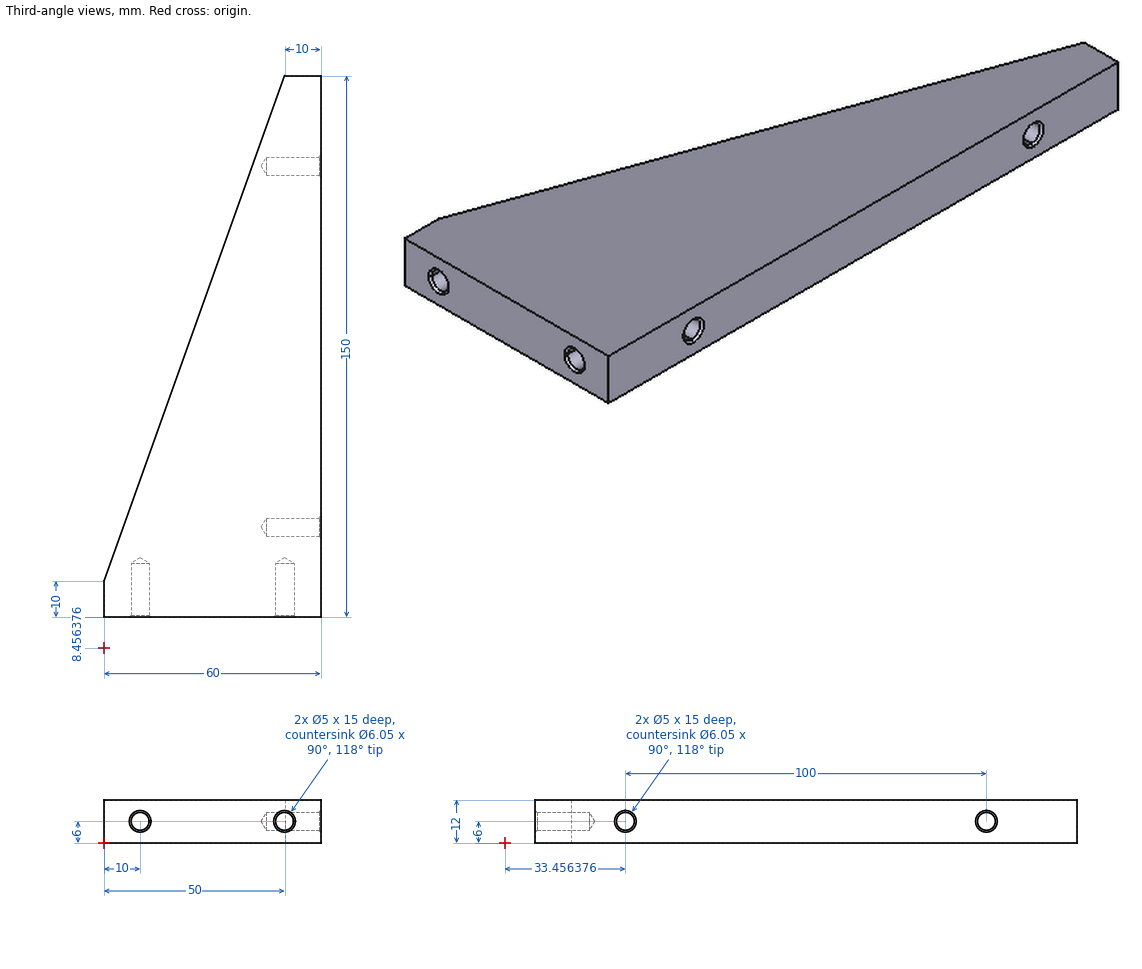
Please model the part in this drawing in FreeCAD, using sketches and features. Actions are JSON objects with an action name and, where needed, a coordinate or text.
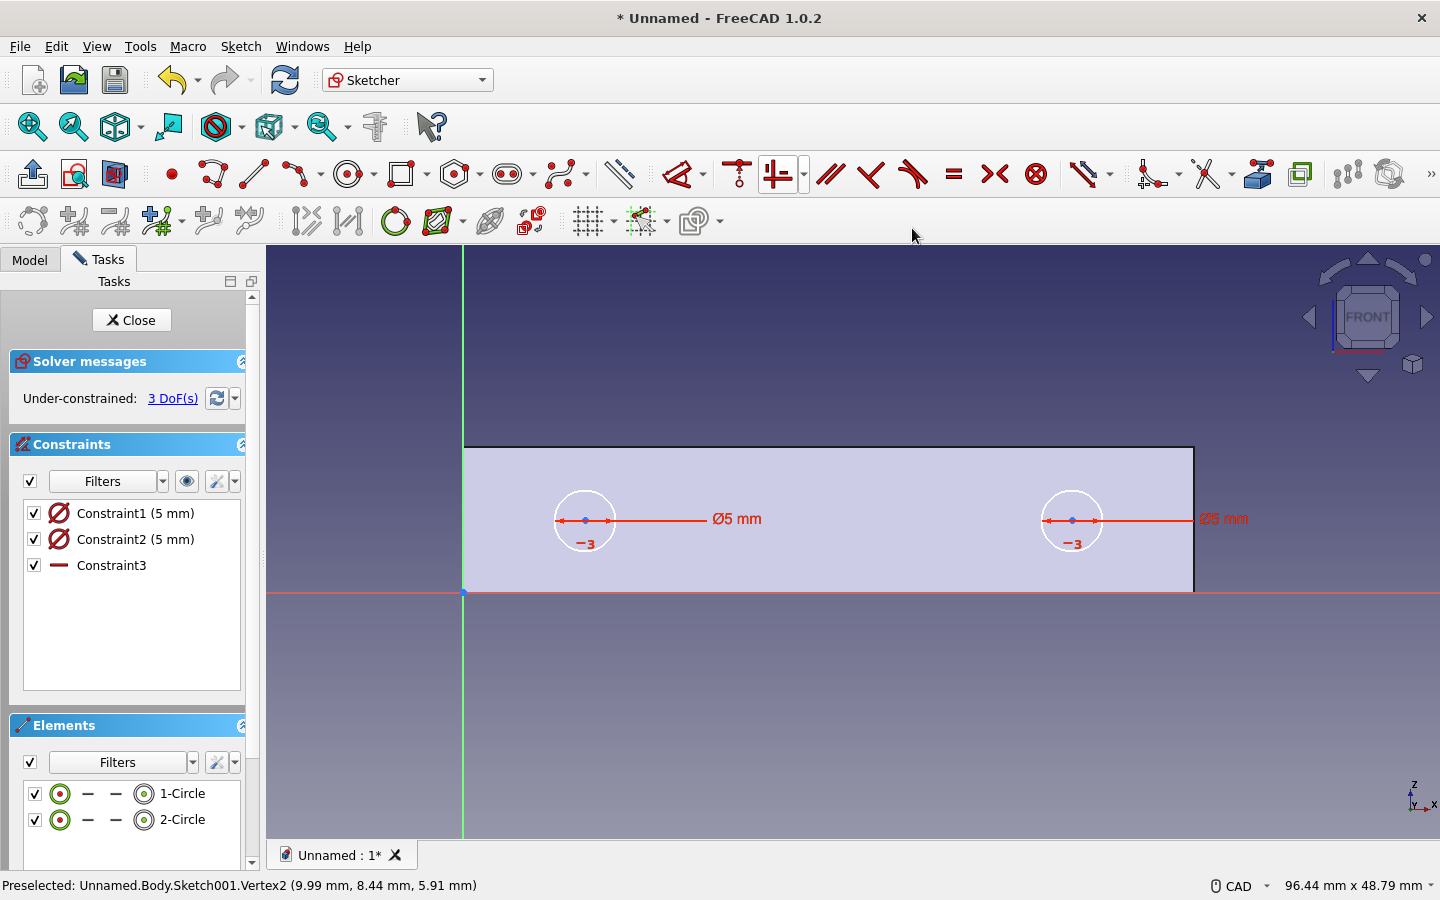
{"action": "left_click", "coordinate": [676, 174]}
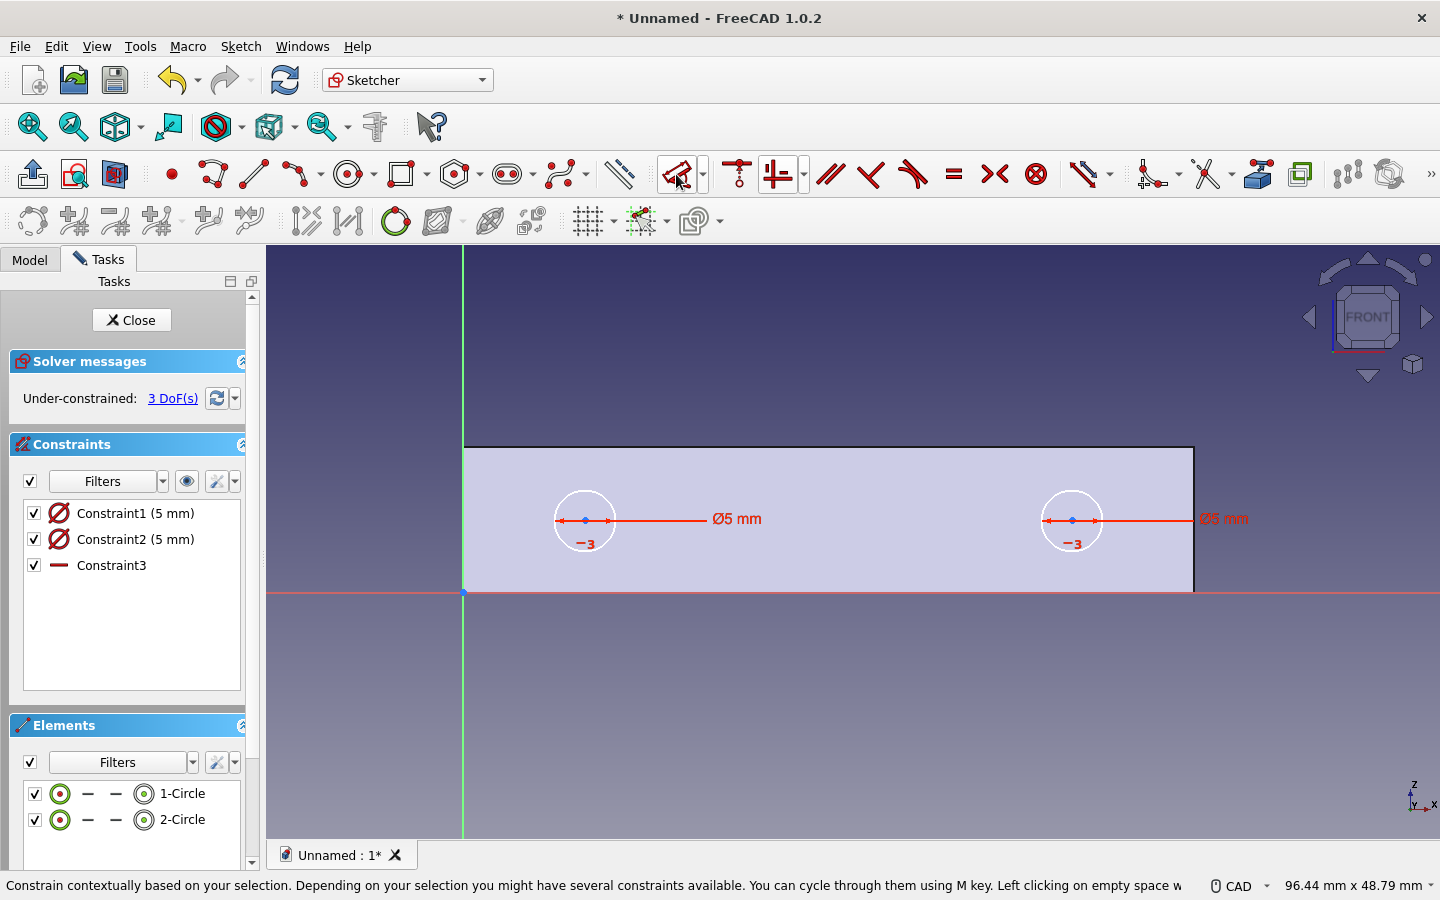
{"action": "left_click", "coordinate": [1072, 521]}
{"action": "left_click", "coordinate": [429, 557]}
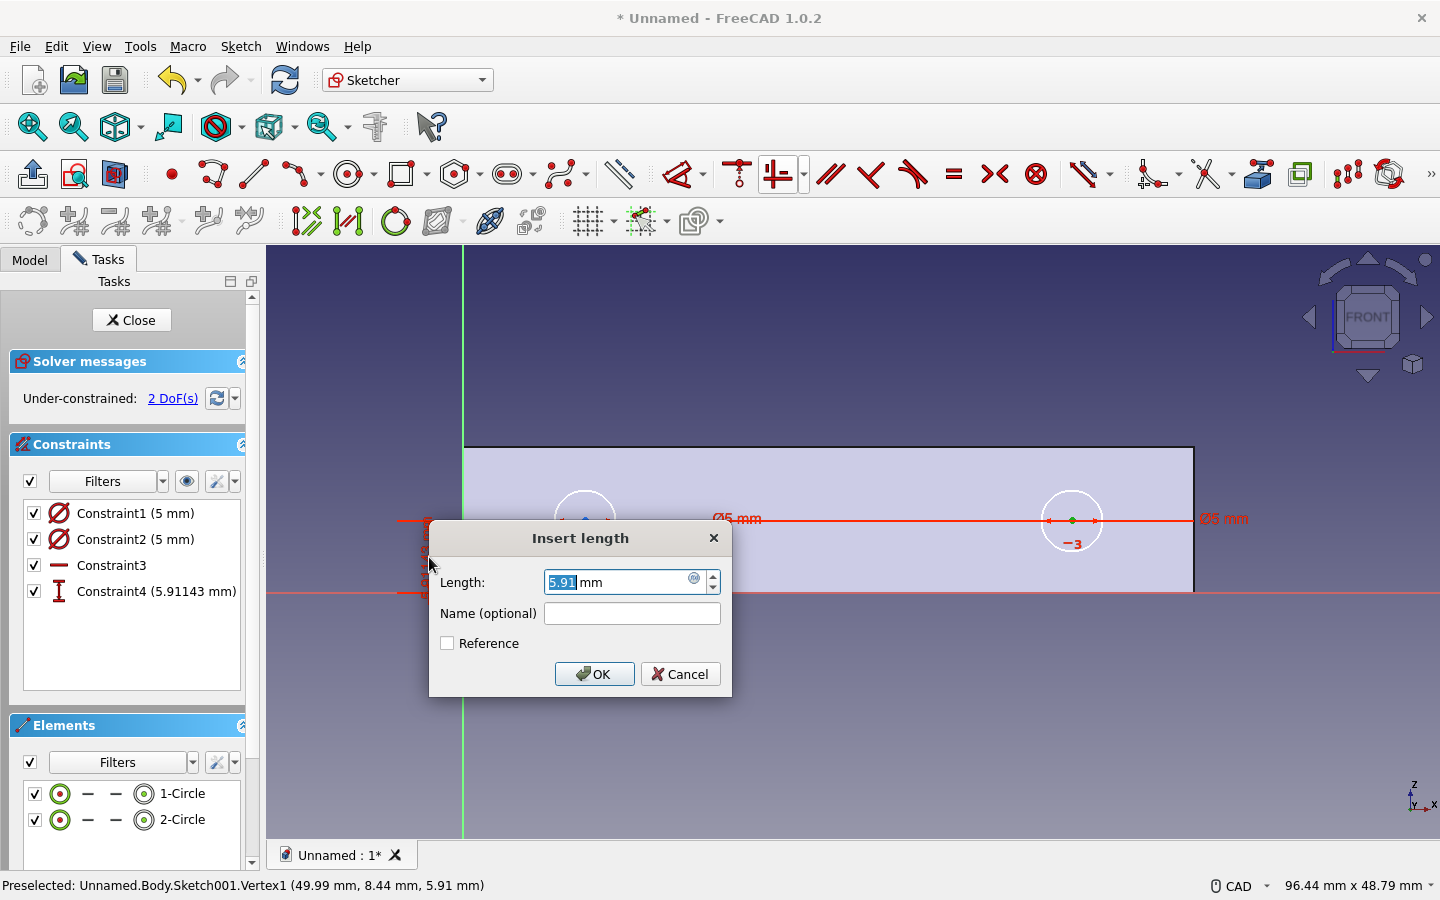
{"action": "type", "text": "6"}
{"action": "key", "text": "Return"}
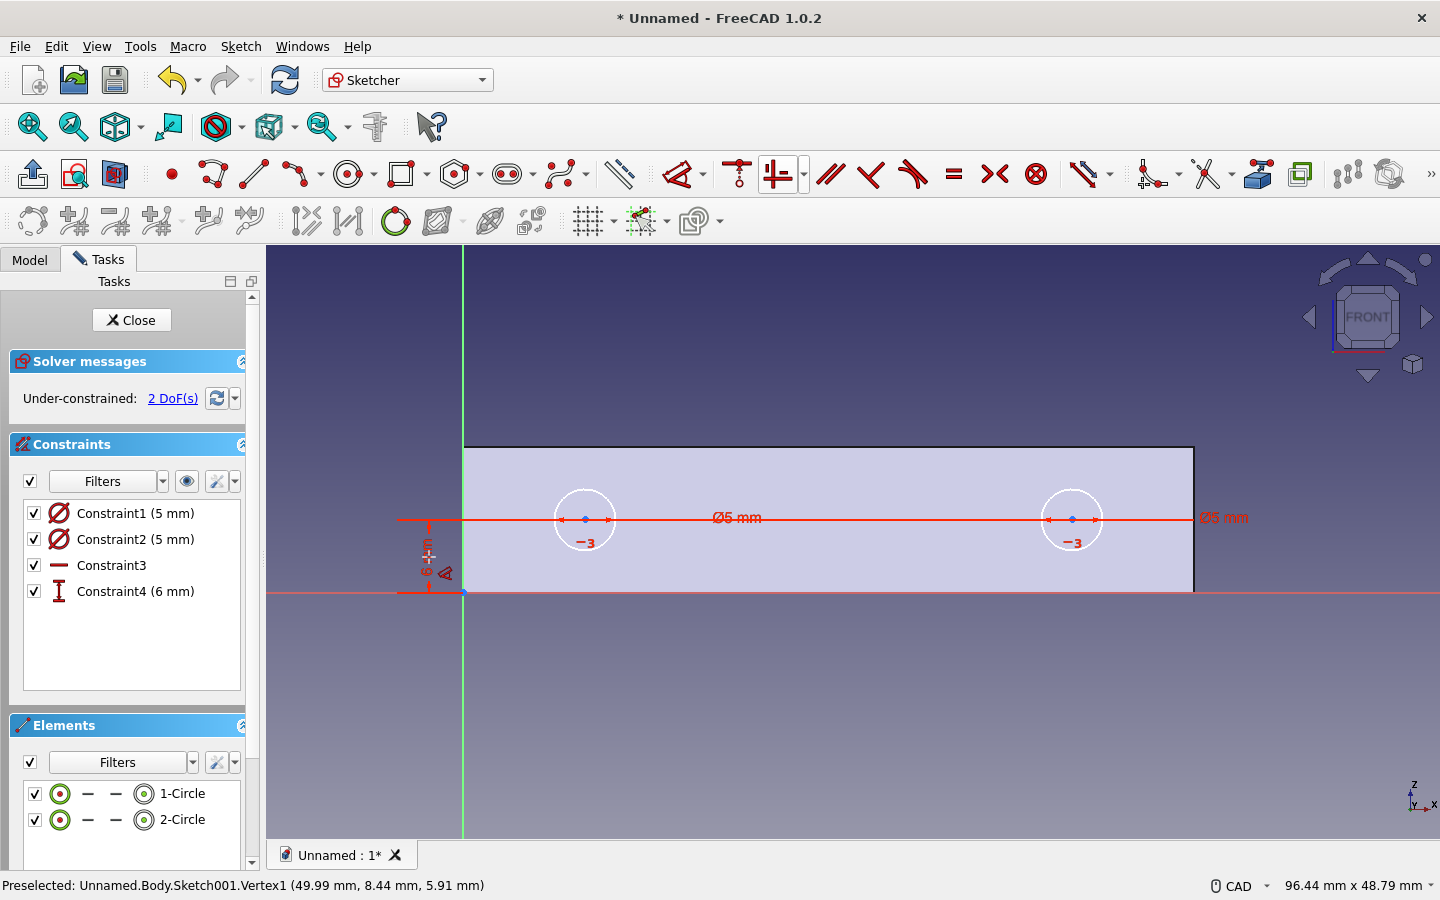
{"action": "left_click", "coordinate": [1072, 520]}
{"action": "left_click", "coordinate": [768, 627]}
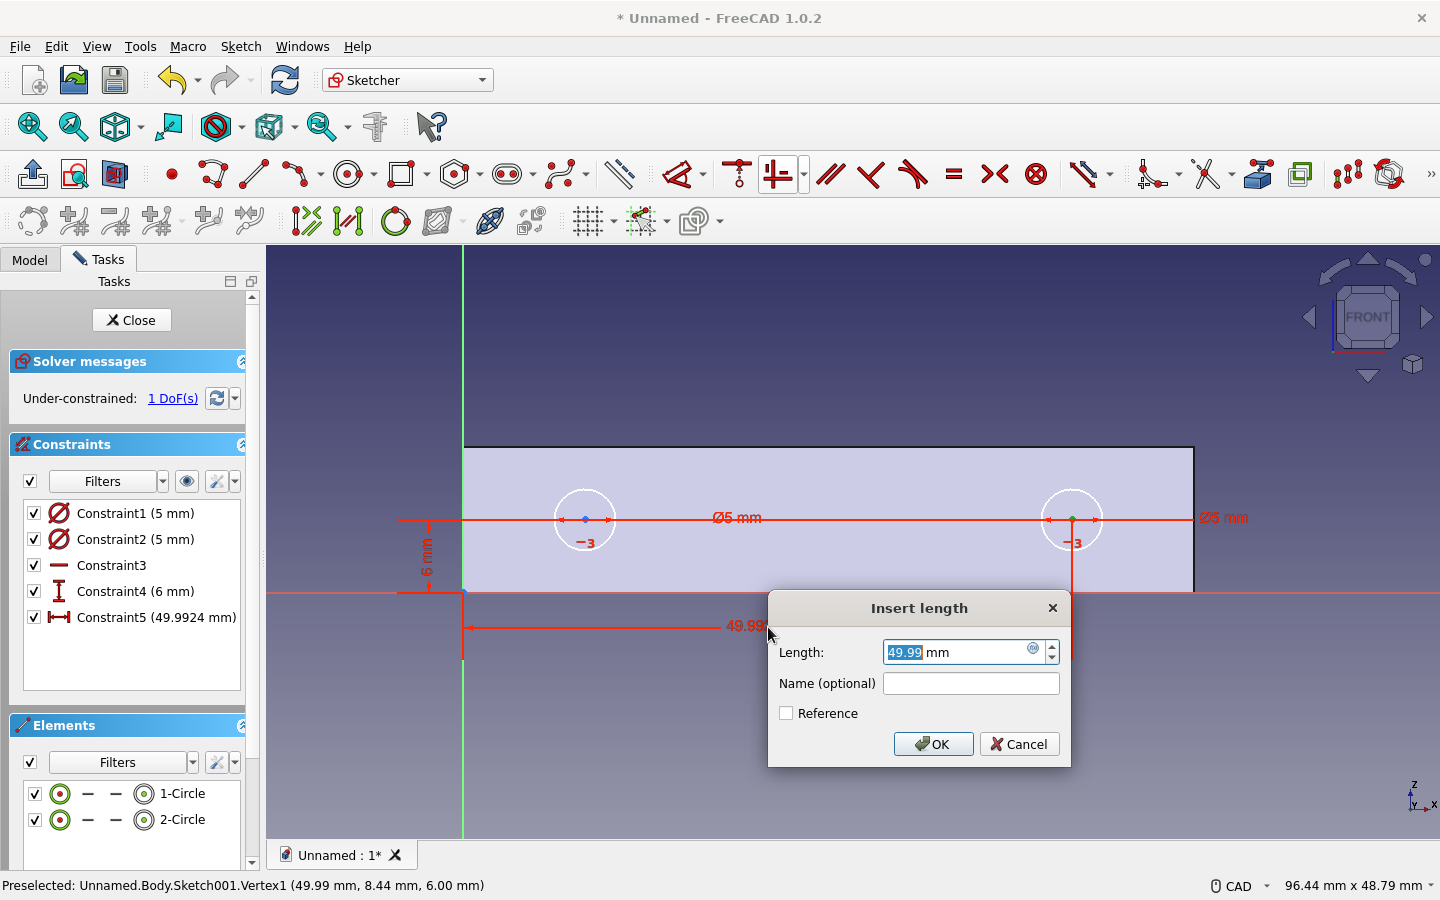
{"action": "type", "text": "50"}
{"action": "key", "text": "Return"}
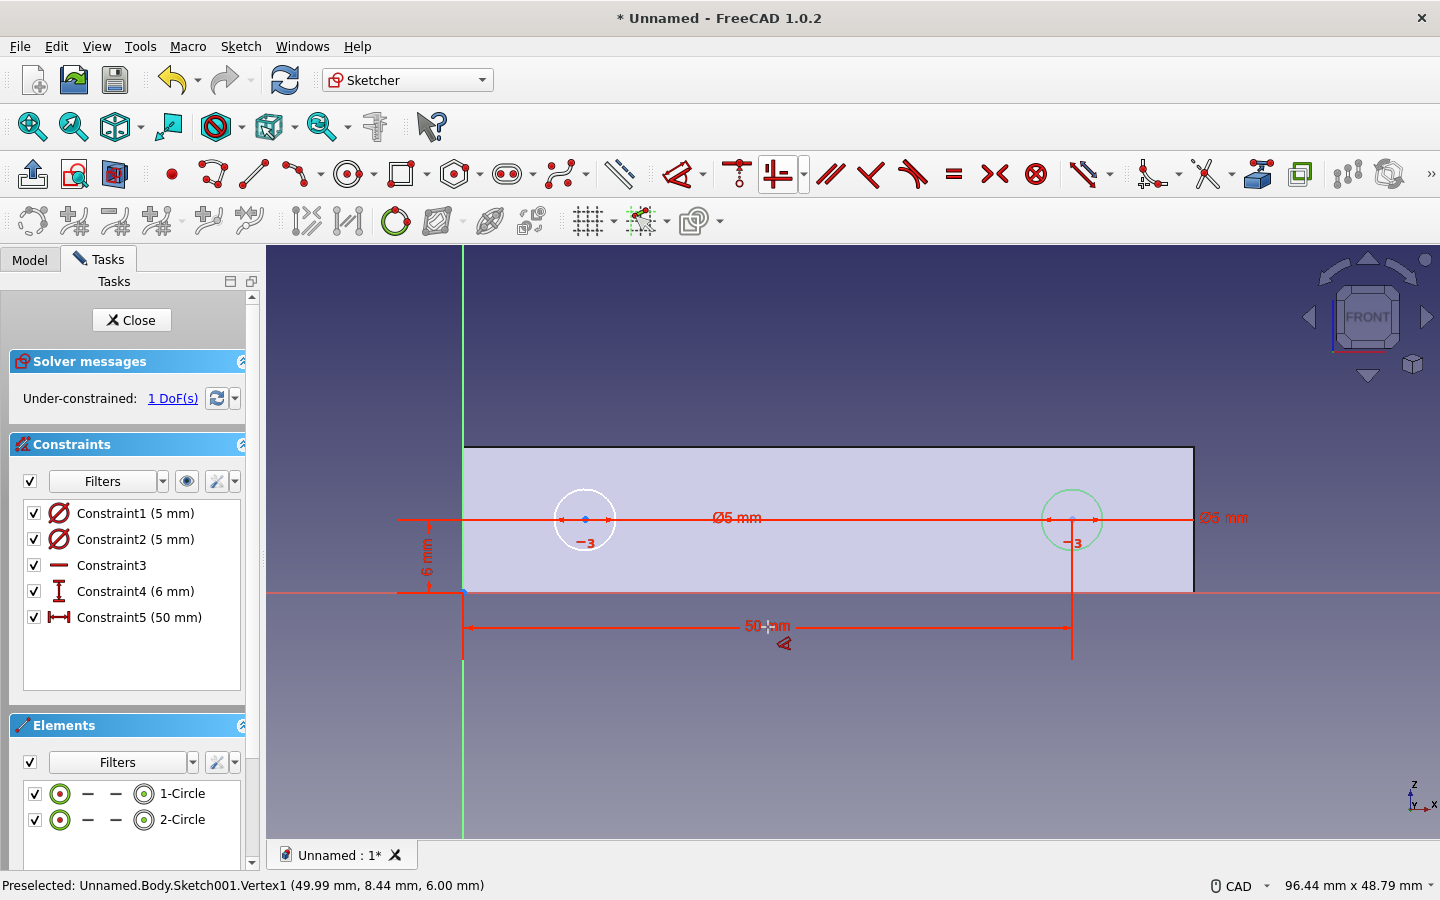
{"action": "left_click", "coordinate": [585, 520]}
{"action": "left_click", "coordinate": [524, 627]}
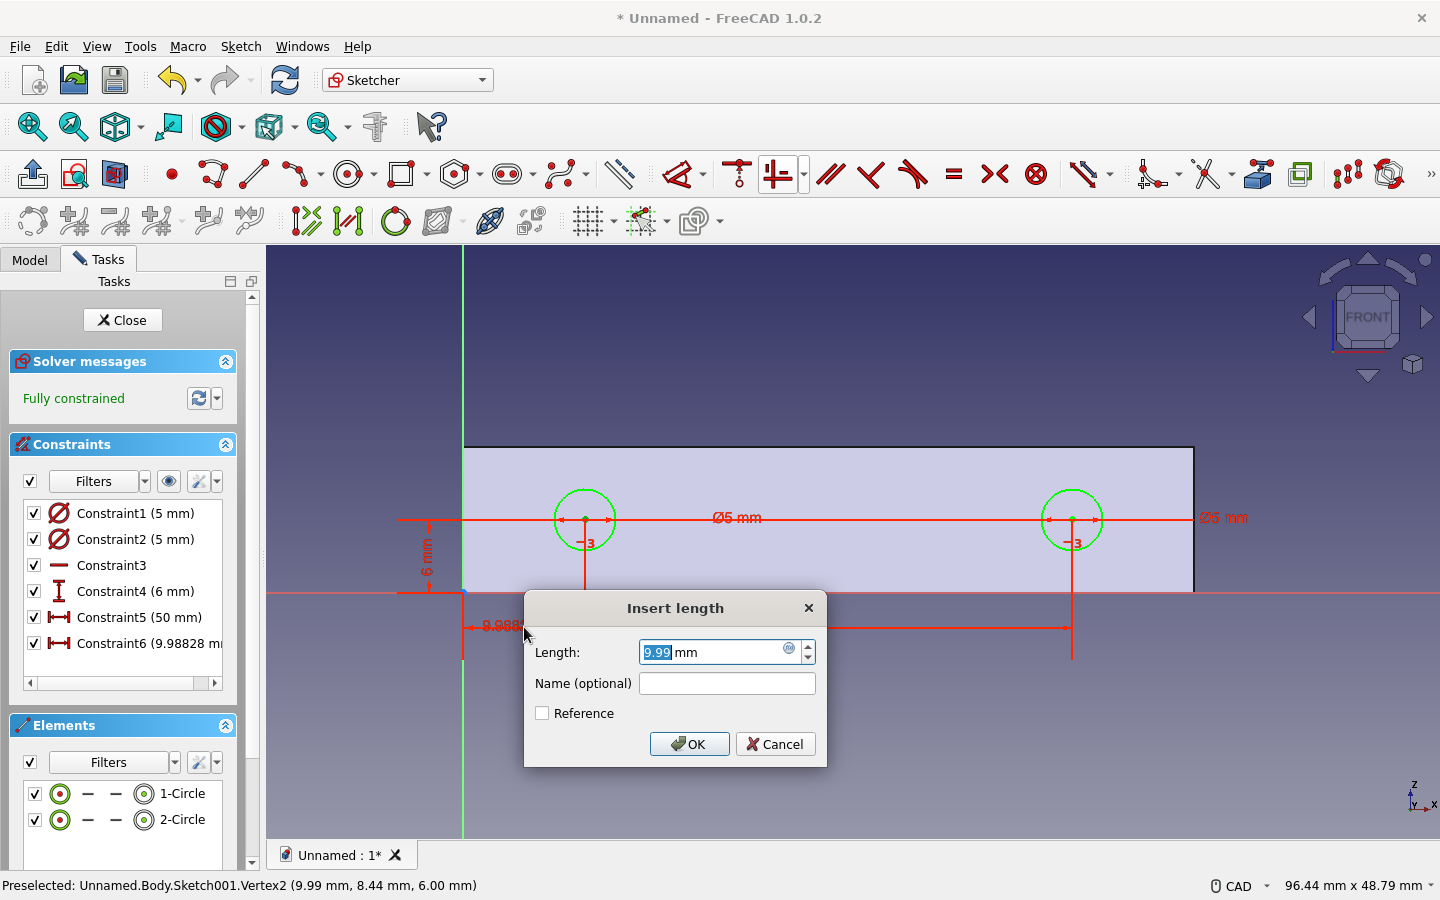
{"action": "type", "text": "10"}
{"action": "key", "text": "Return"}
{"action": "key", "text": "Escape"}